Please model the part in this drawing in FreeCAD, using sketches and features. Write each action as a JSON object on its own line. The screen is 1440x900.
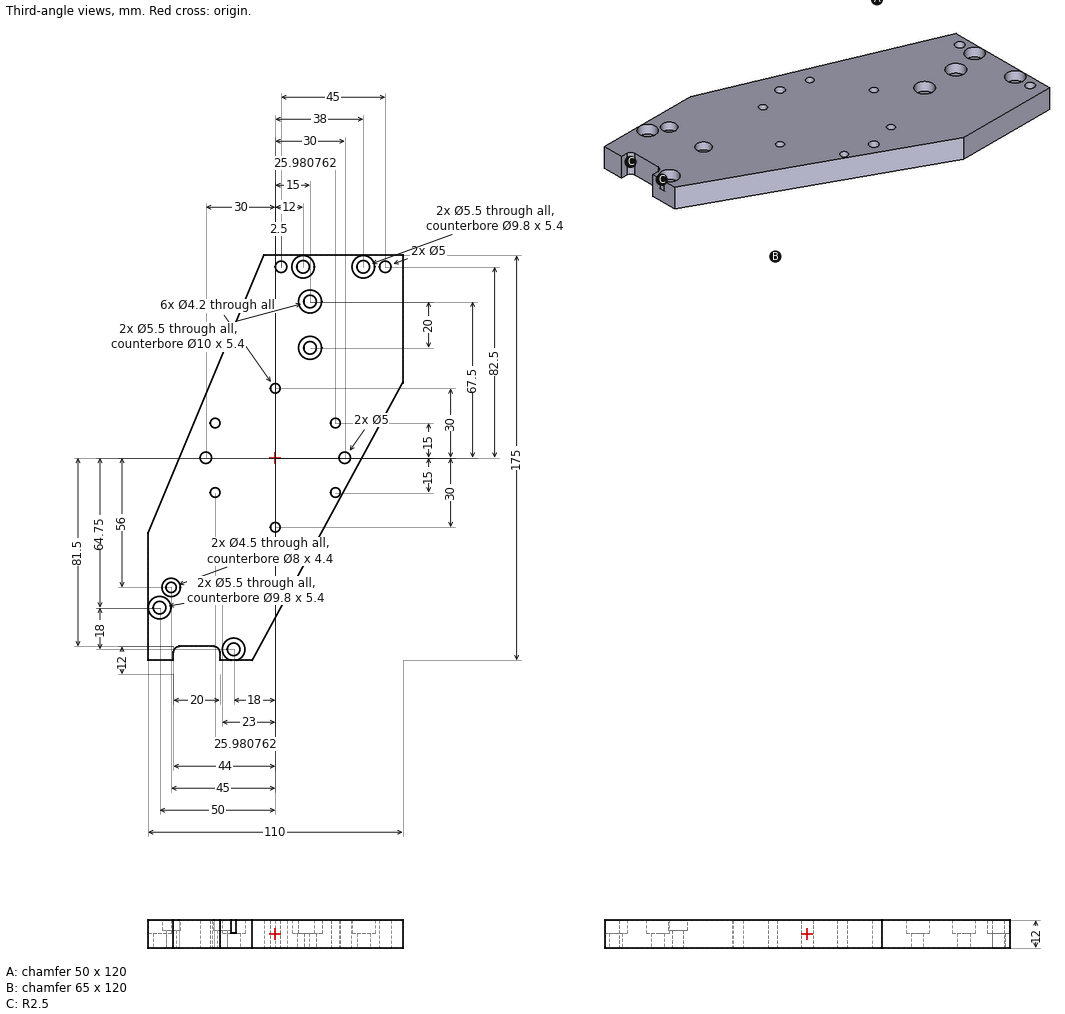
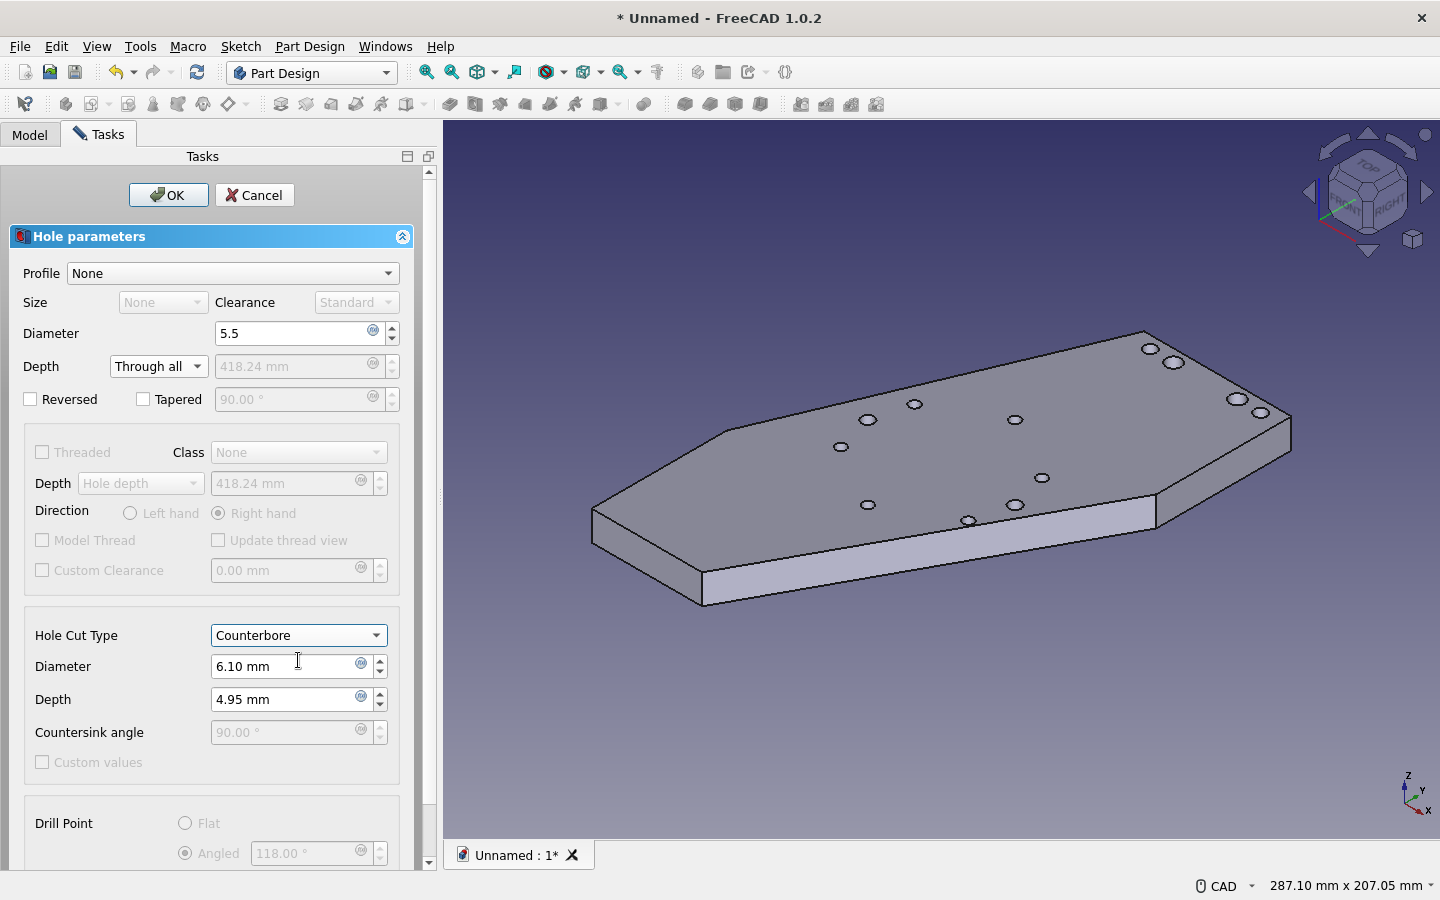
{"action": "triple_click", "coordinate": [292, 666]}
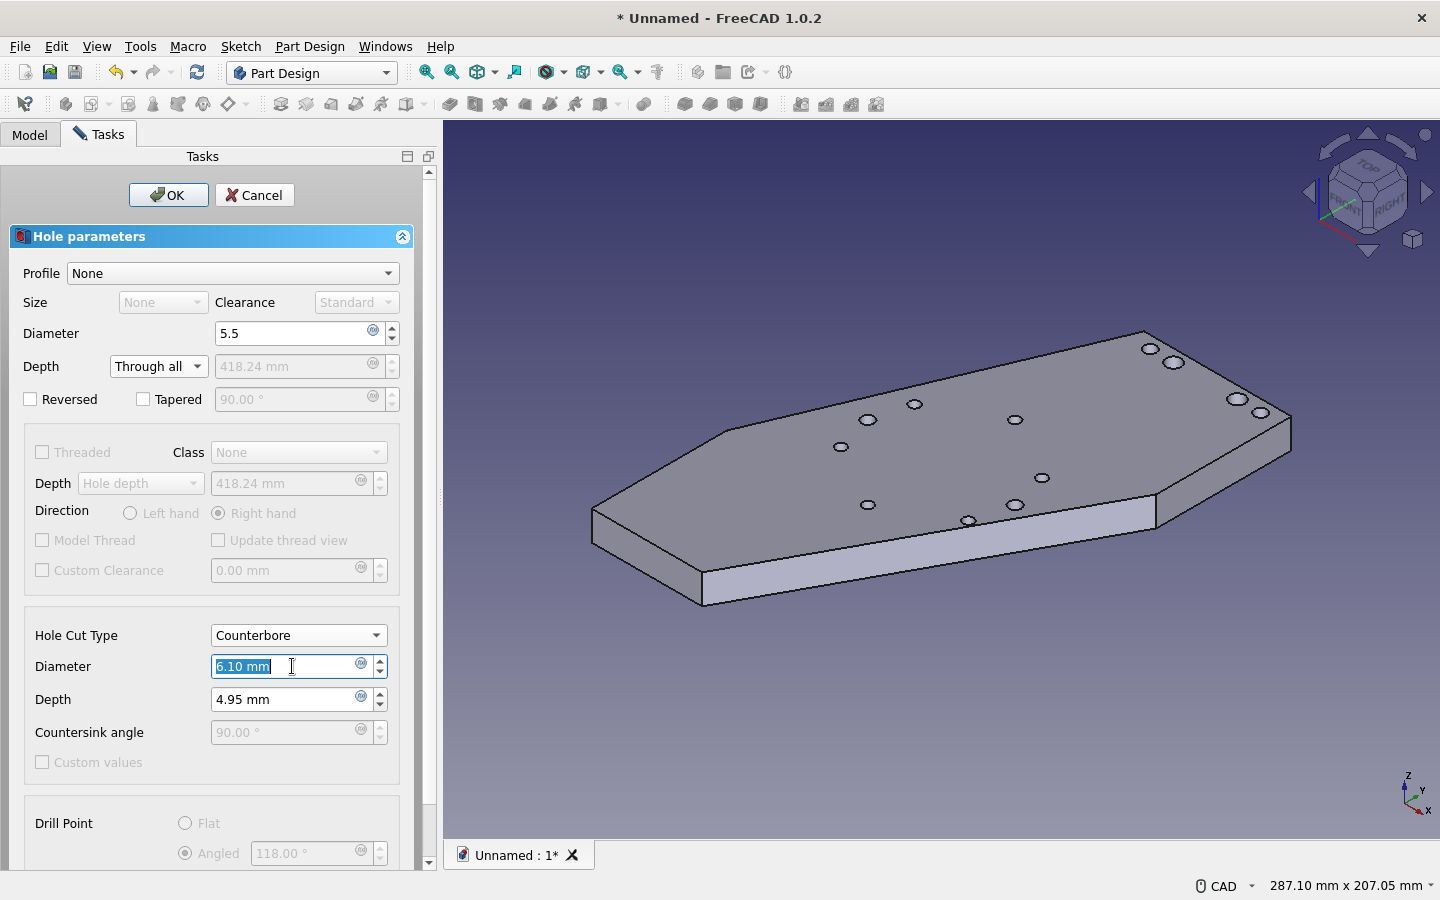
{"action": "type", "text": "9.8"}
{"action": "key", "text": "Tab"}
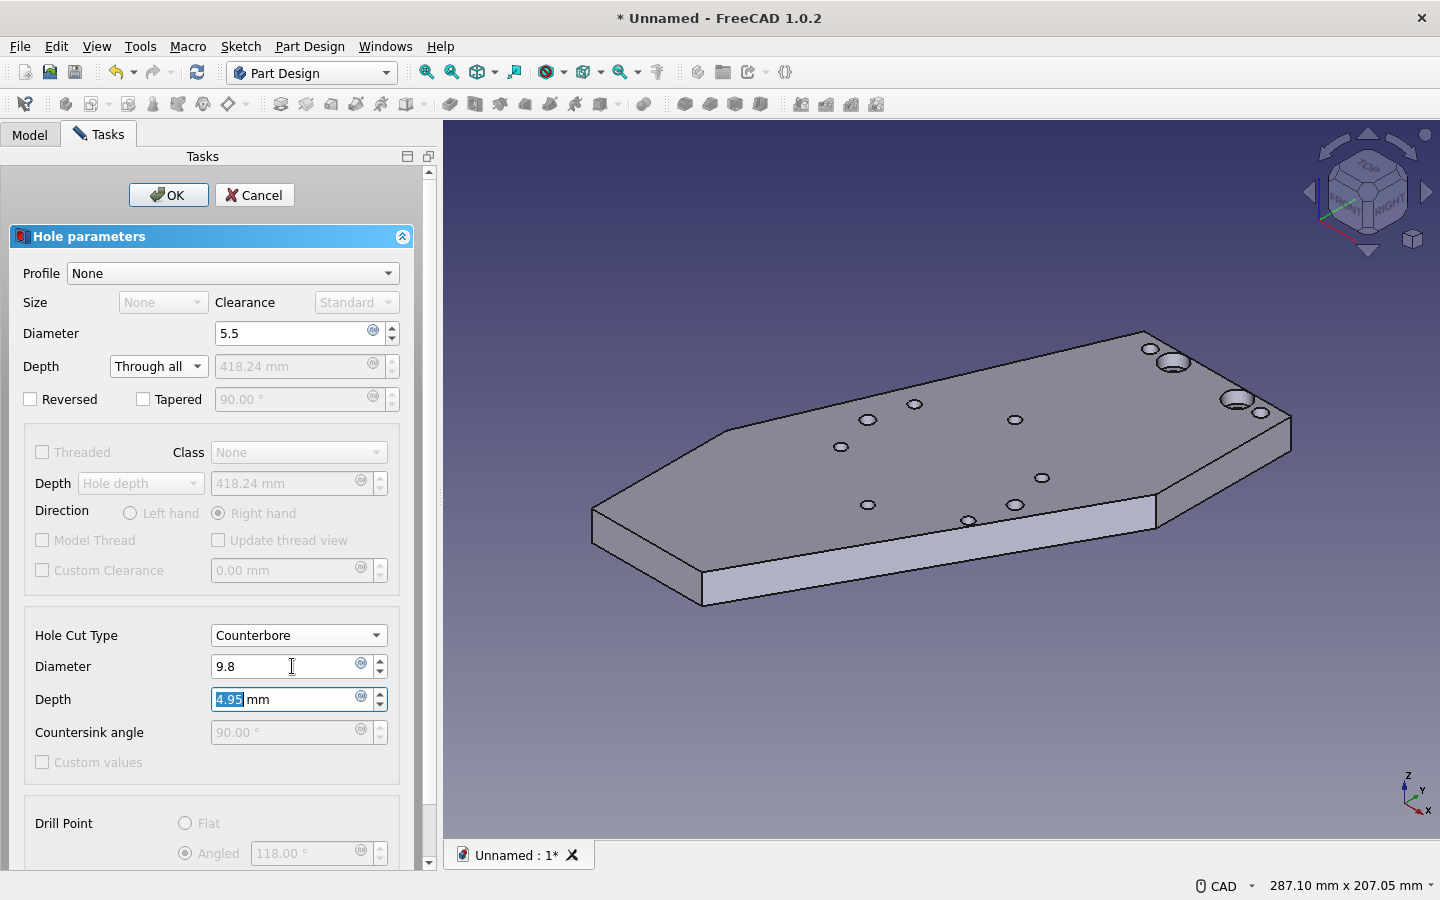
{"action": "type", "text": "5.4"}
{"action": "key", "text": "Tab"}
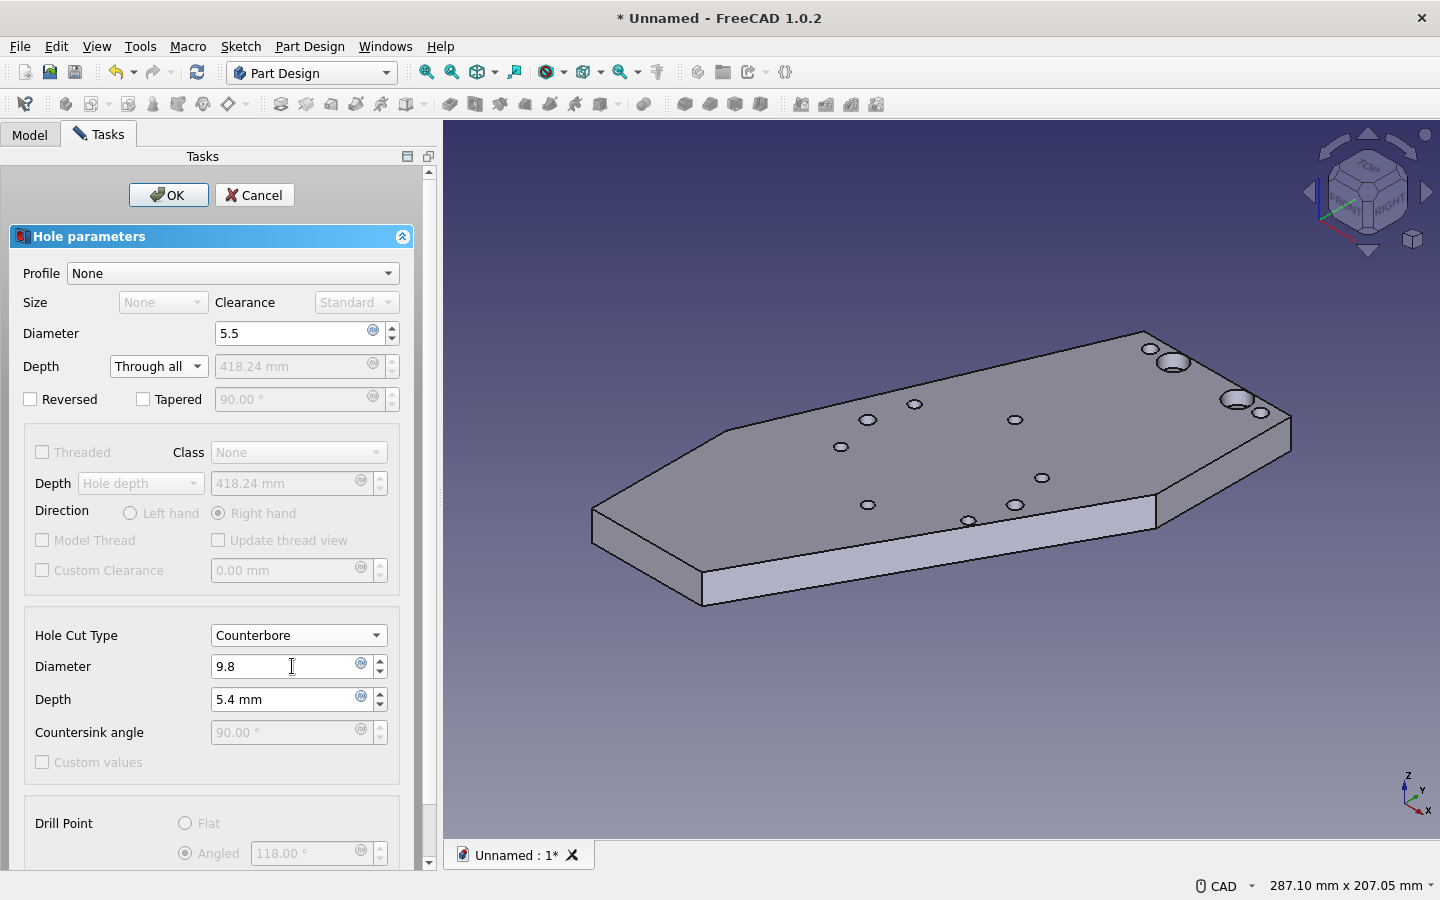
{"action": "left_click", "coordinate": [169, 195]}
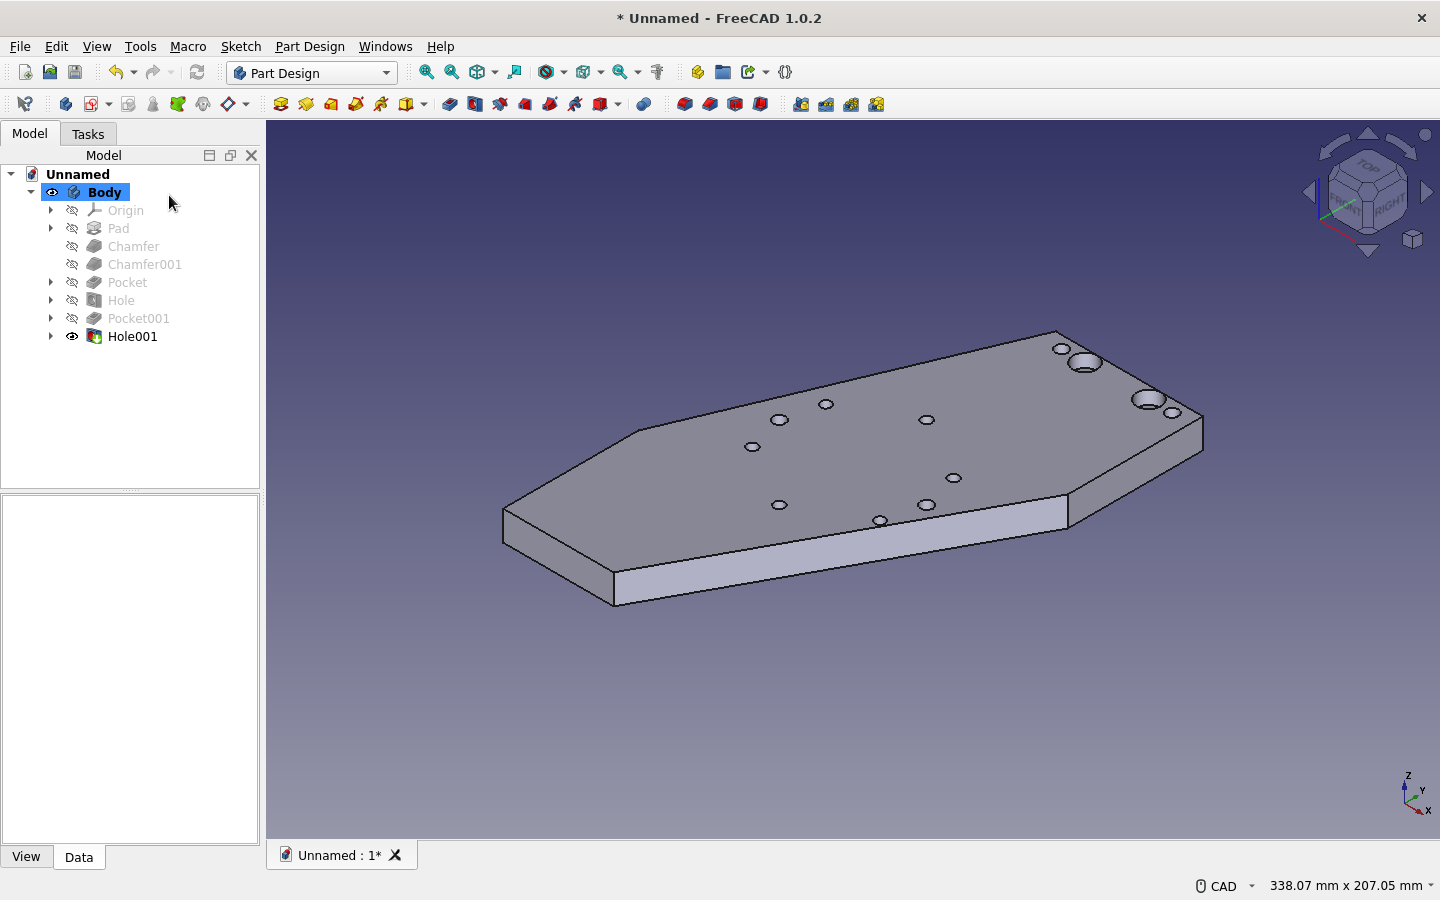
{"action": "left_click", "coordinate": [853, 461]}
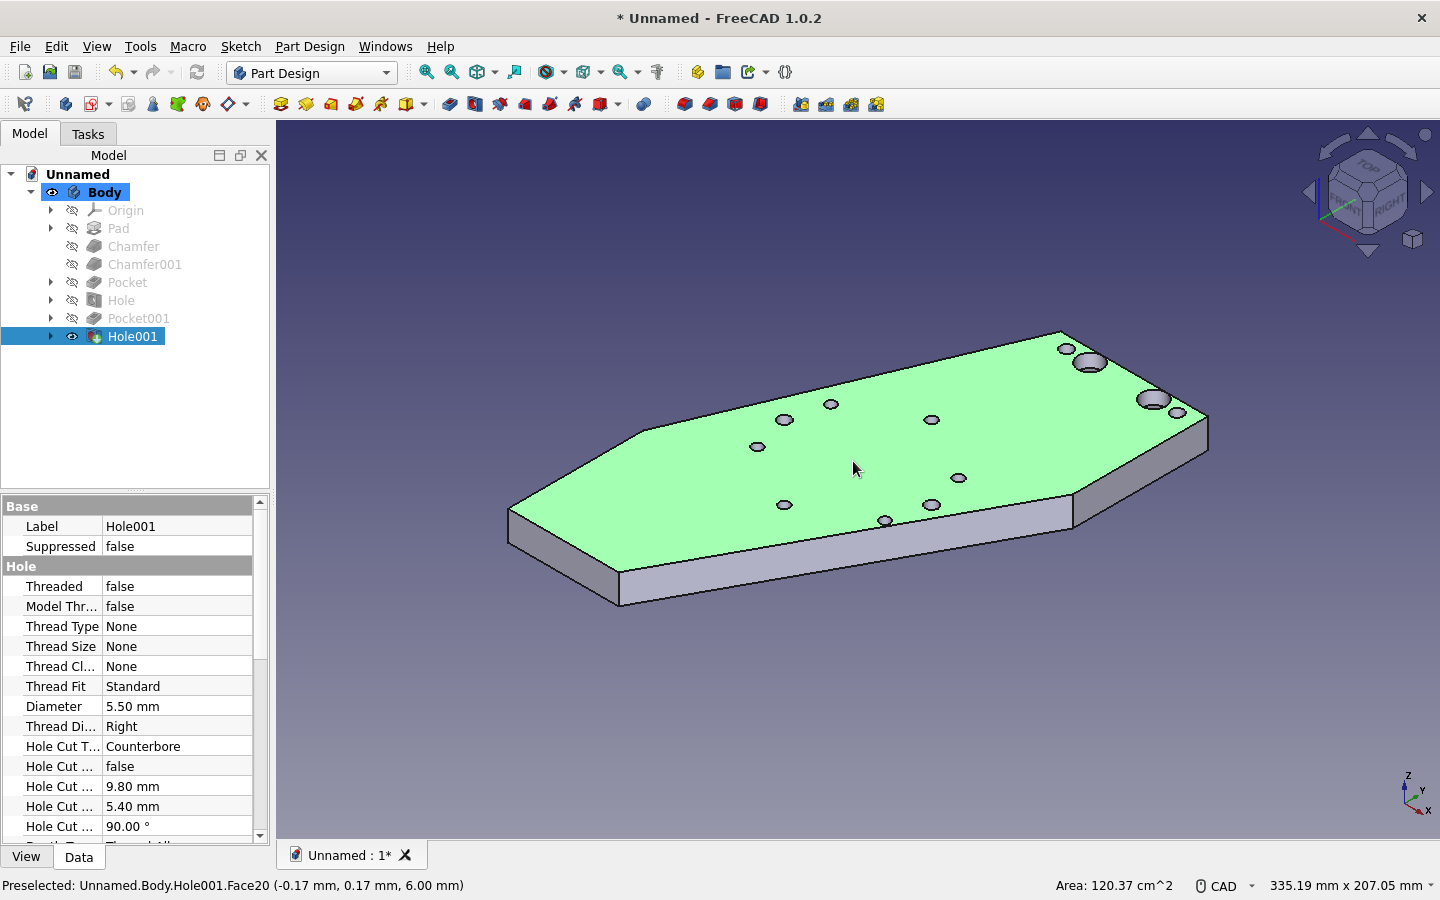
{"action": "left_click", "coordinate": [90, 104]}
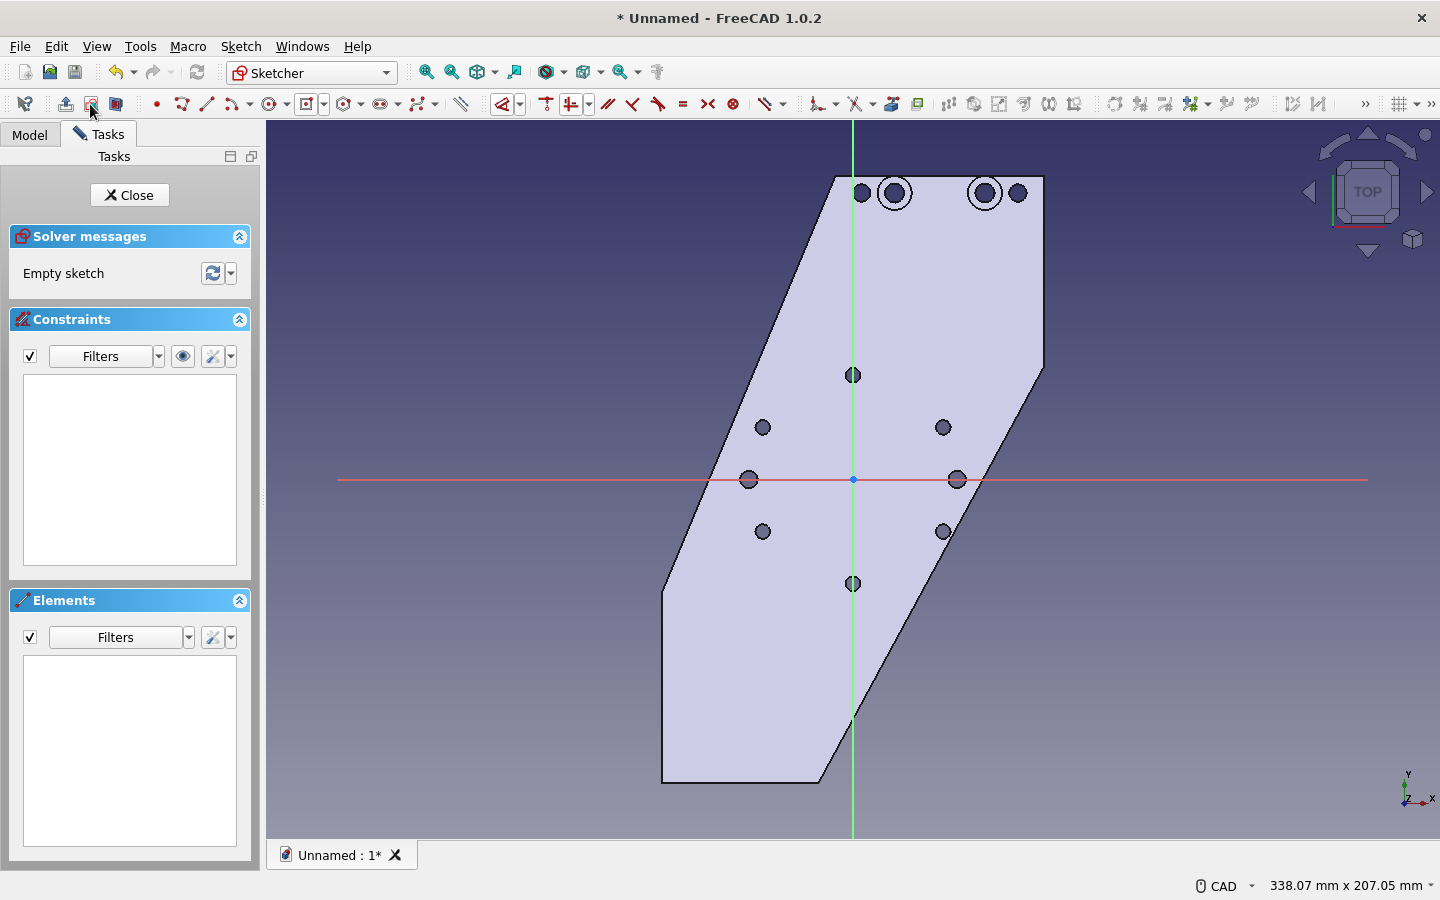
{"action": "scroll", "coordinate": [936, 229], "scroll_direction": "up", "scroll_amount": 8}